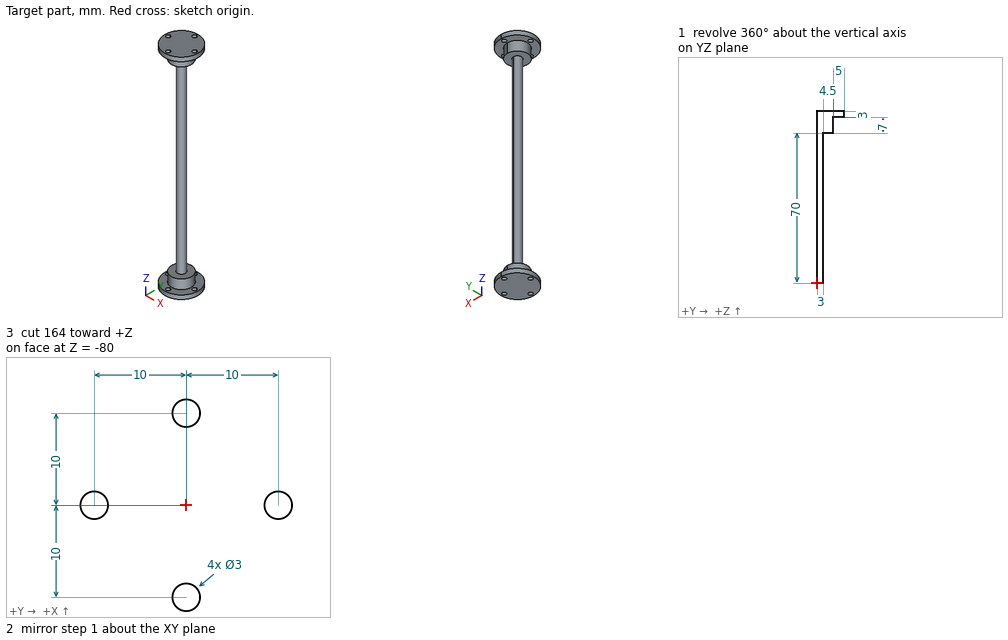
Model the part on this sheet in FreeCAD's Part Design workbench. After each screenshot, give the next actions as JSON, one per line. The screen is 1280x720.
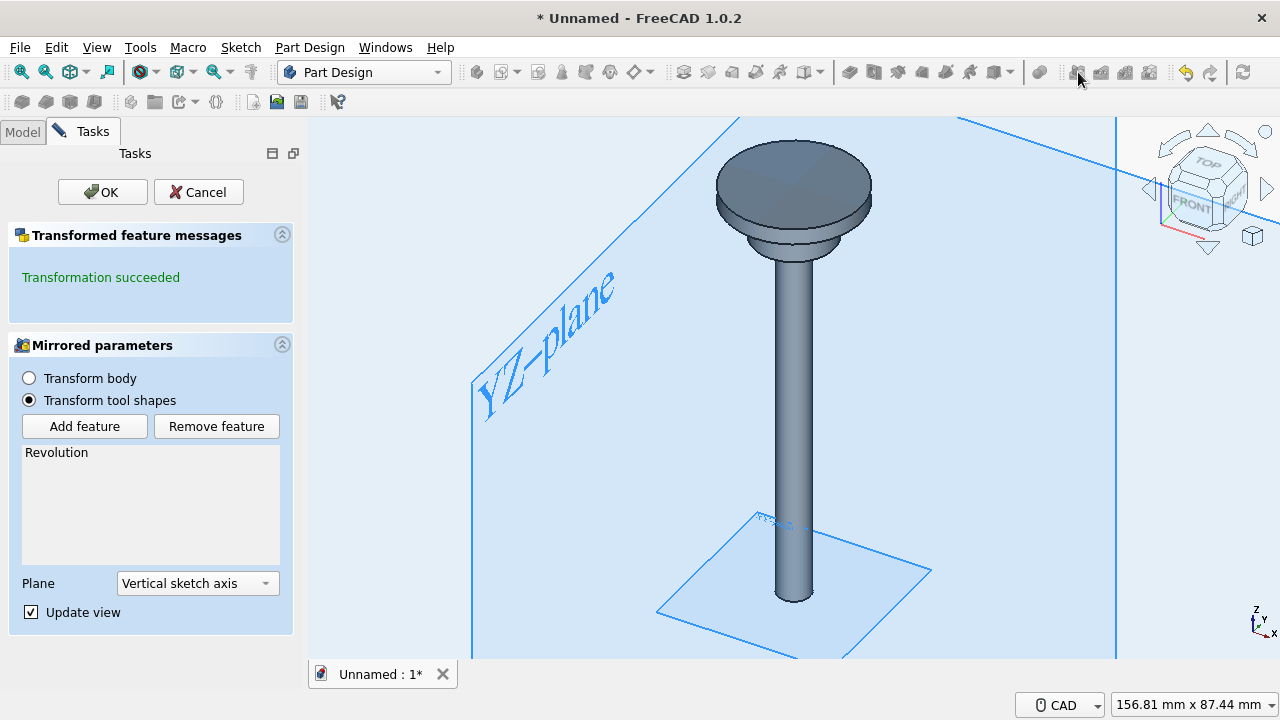
{"action": "left_click", "coordinate": [198, 584]}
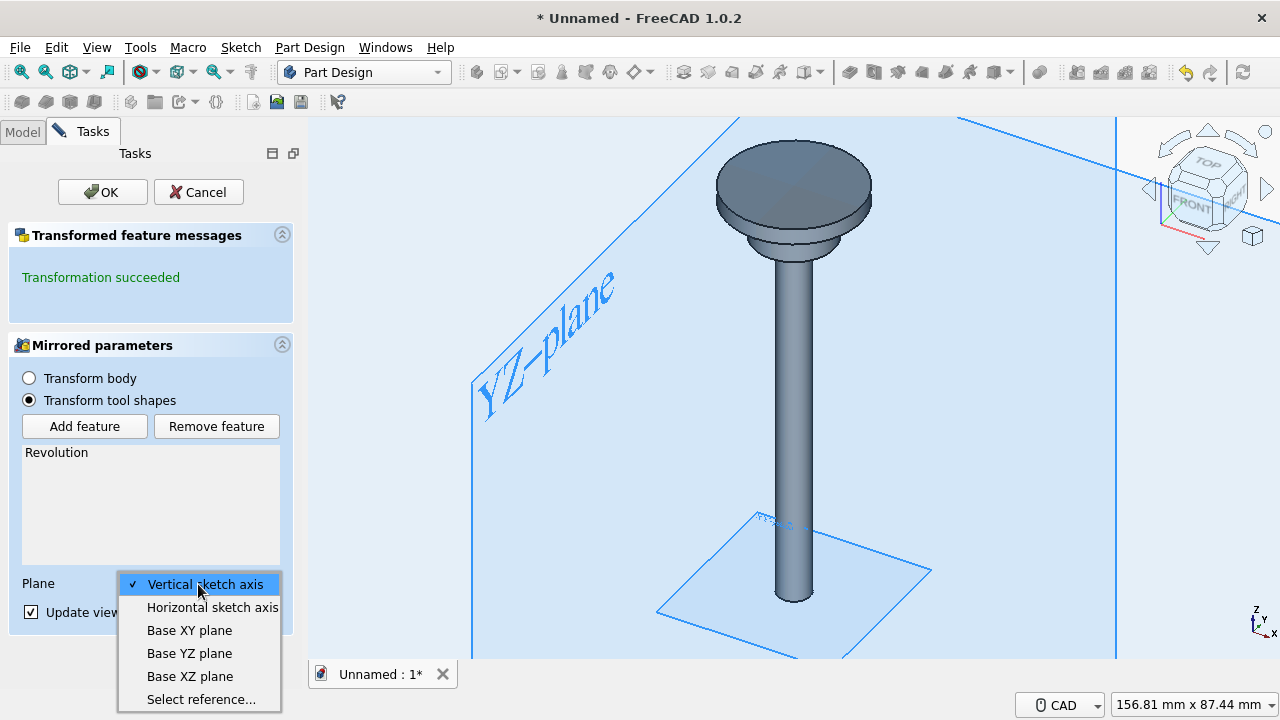
{"action": "left_click", "coordinate": [198, 630]}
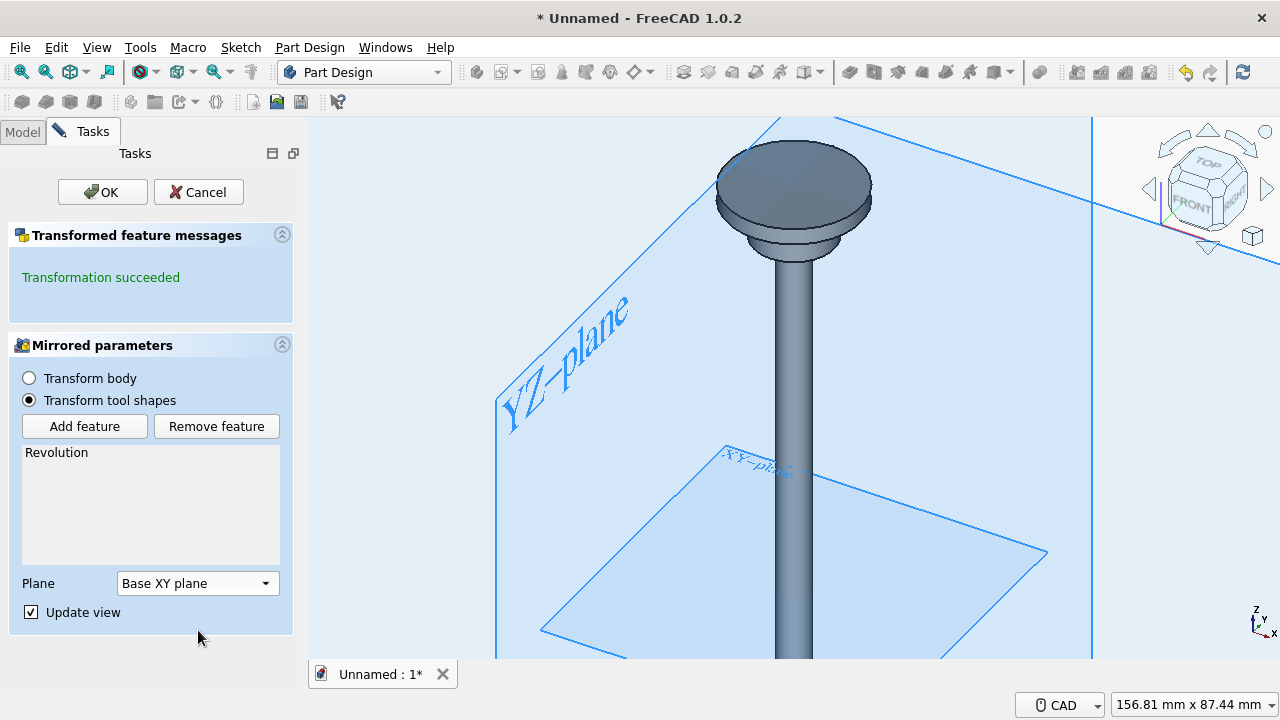
{"action": "left_click", "coordinate": [103, 192]}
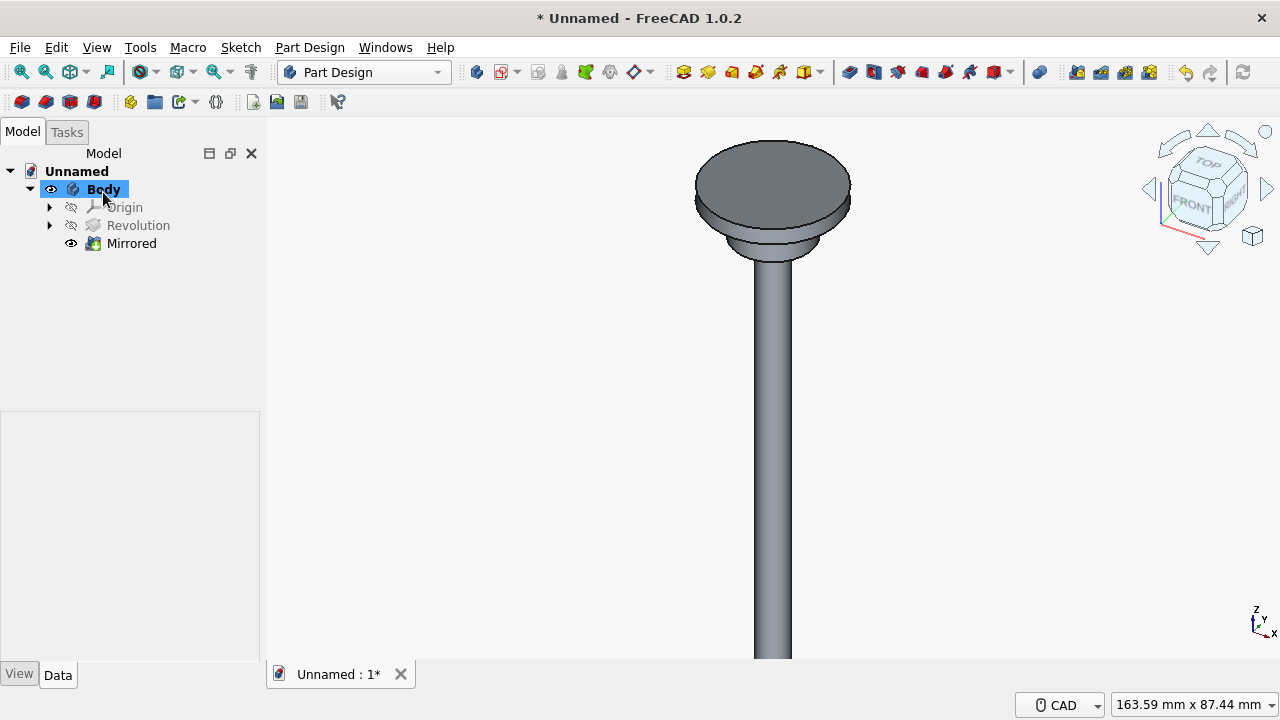
{"action": "left_click", "coordinate": [22, 72]}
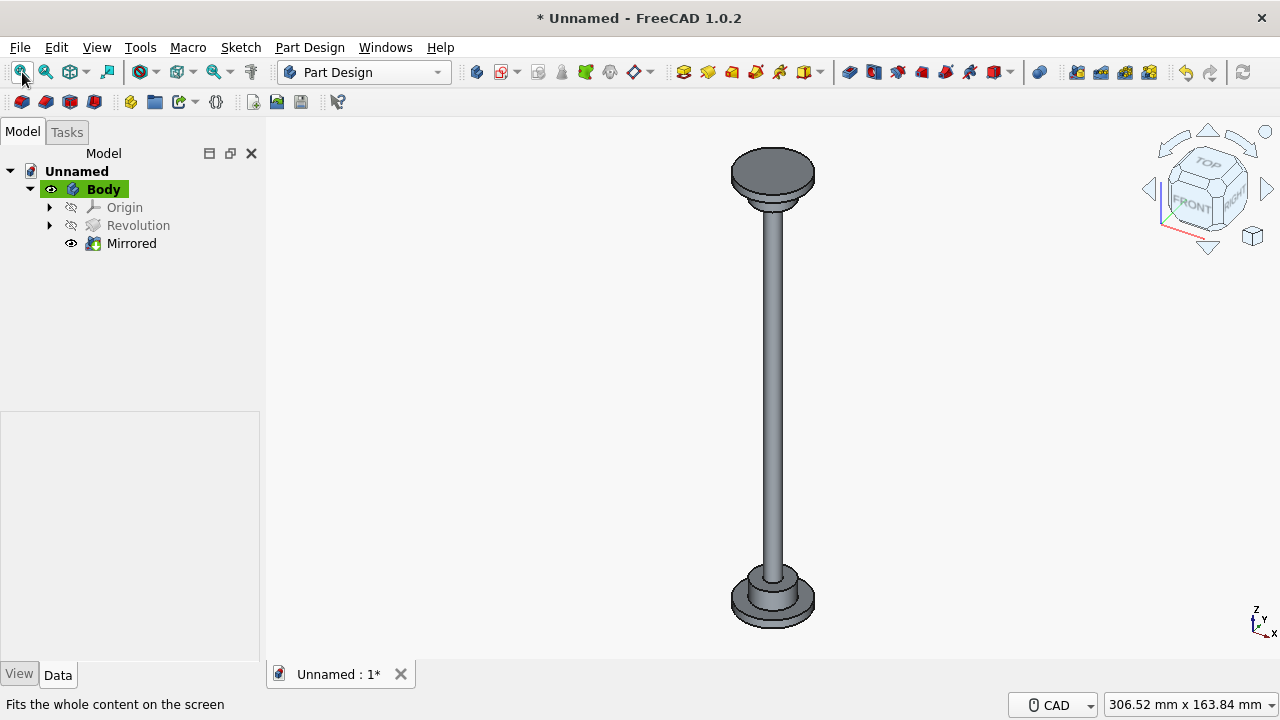
{"action": "key", "text": "5"}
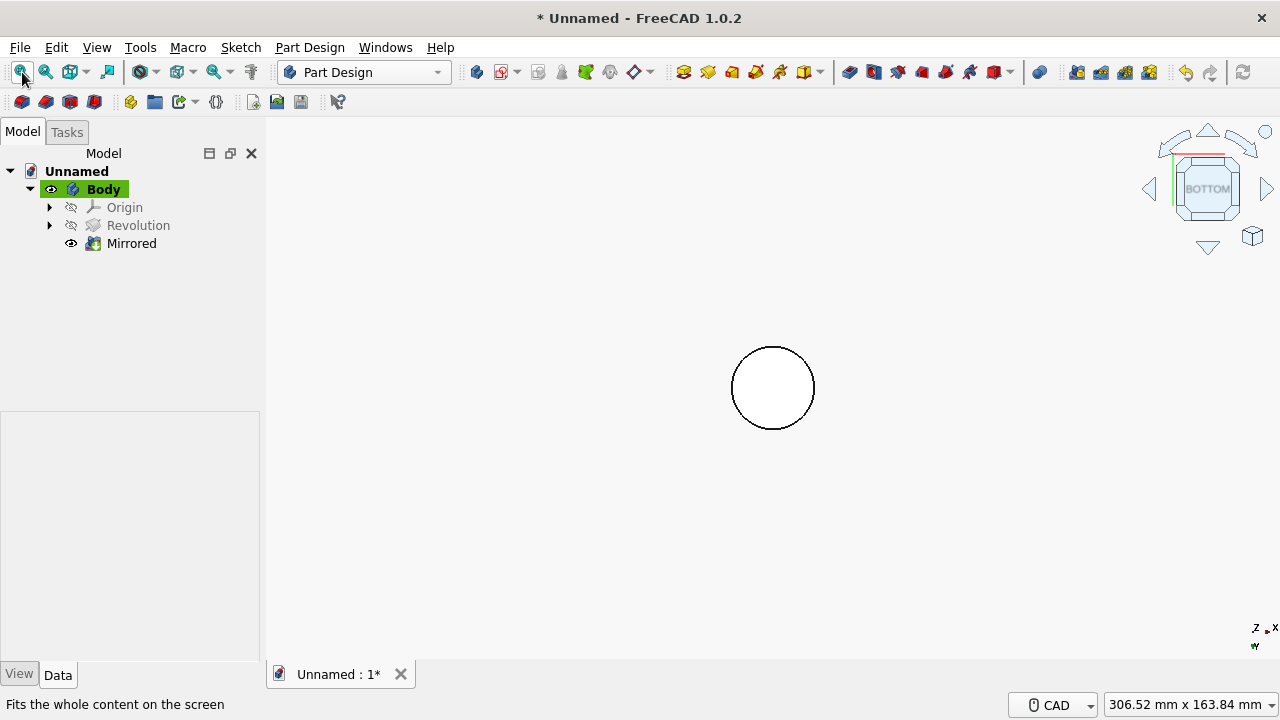
{"action": "left_click", "coordinate": [22, 72]}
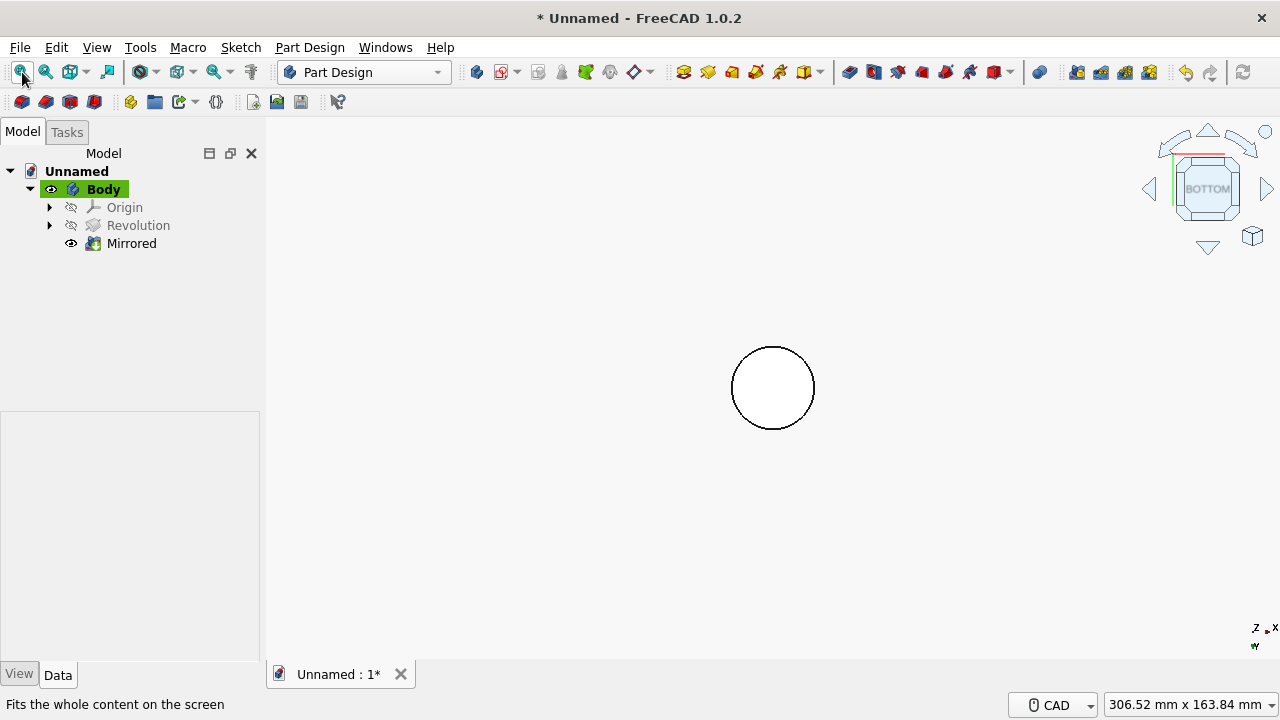
{"action": "left_click", "coordinate": [773, 387]}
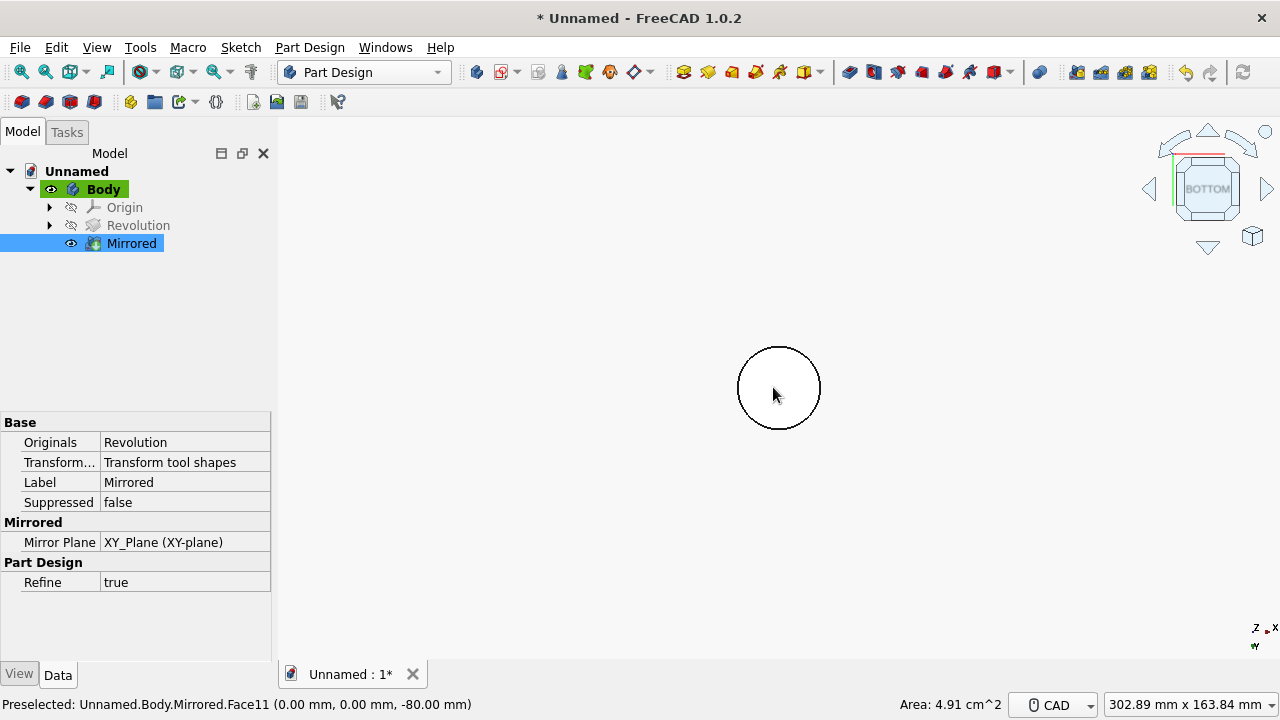
{"action": "left_click", "coordinate": [502, 72]}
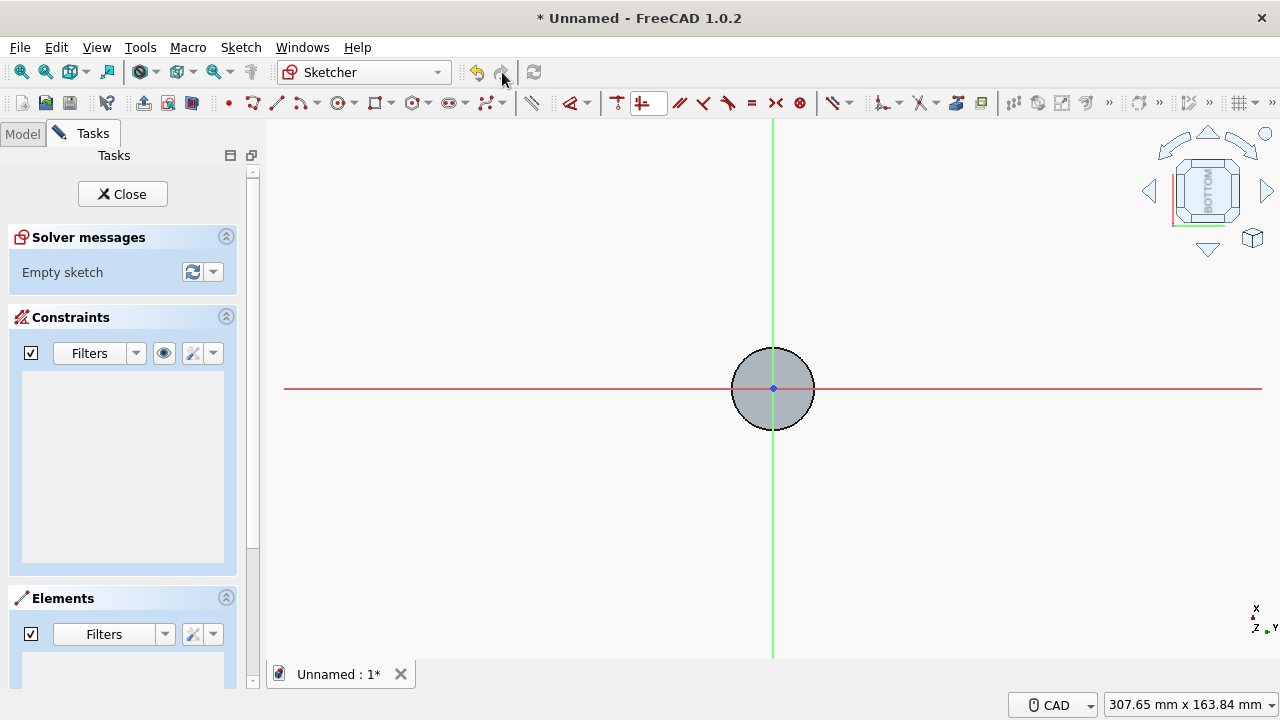
{"action": "scroll", "coordinate": [790, 389], "scroll_direction": "up", "scroll_amount": 8}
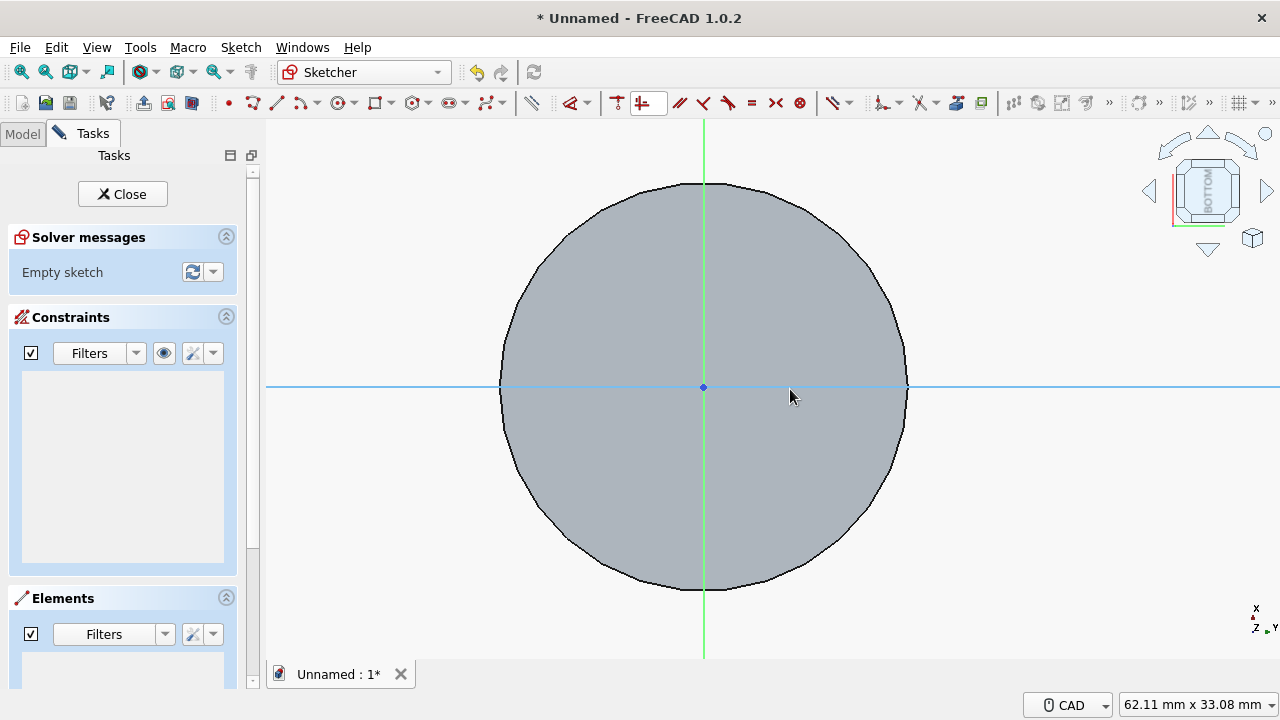
{"action": "left_click", "coordinate": [338, 104]}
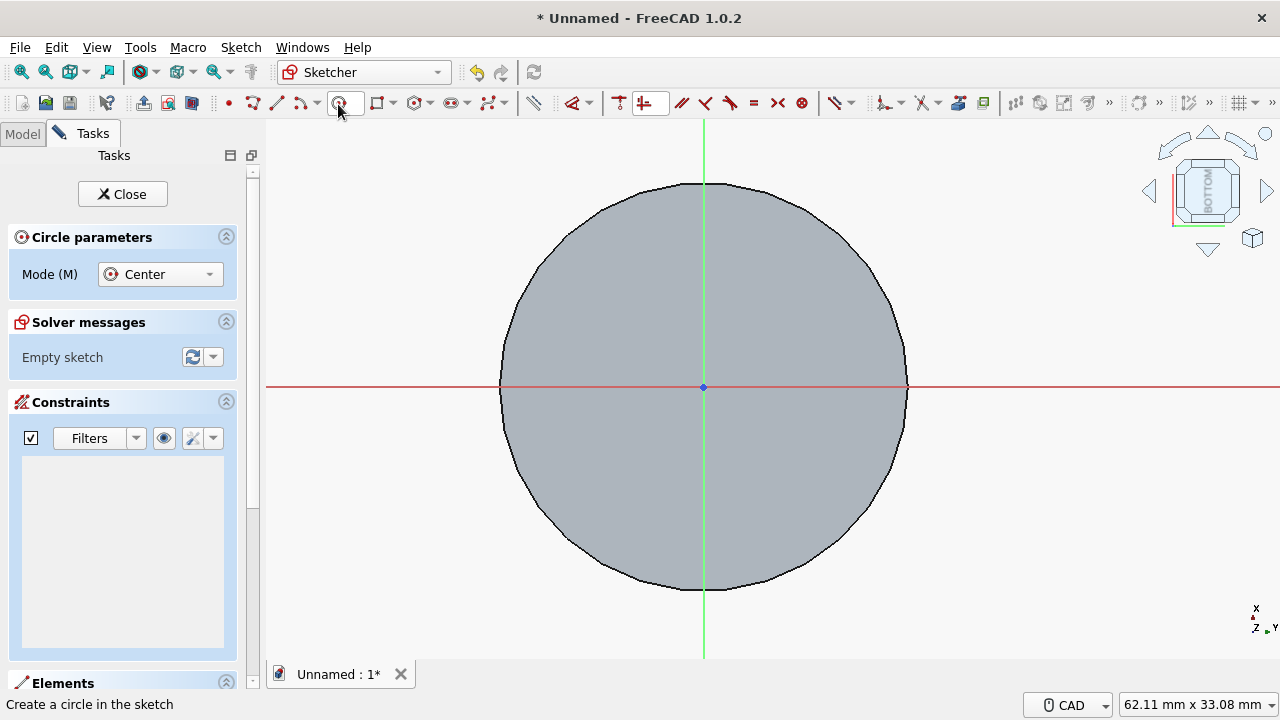
{"action": "left_click", "coordinate": [704, 550]}
{"action": "mouse_move", "coordinate": [721, 533]}